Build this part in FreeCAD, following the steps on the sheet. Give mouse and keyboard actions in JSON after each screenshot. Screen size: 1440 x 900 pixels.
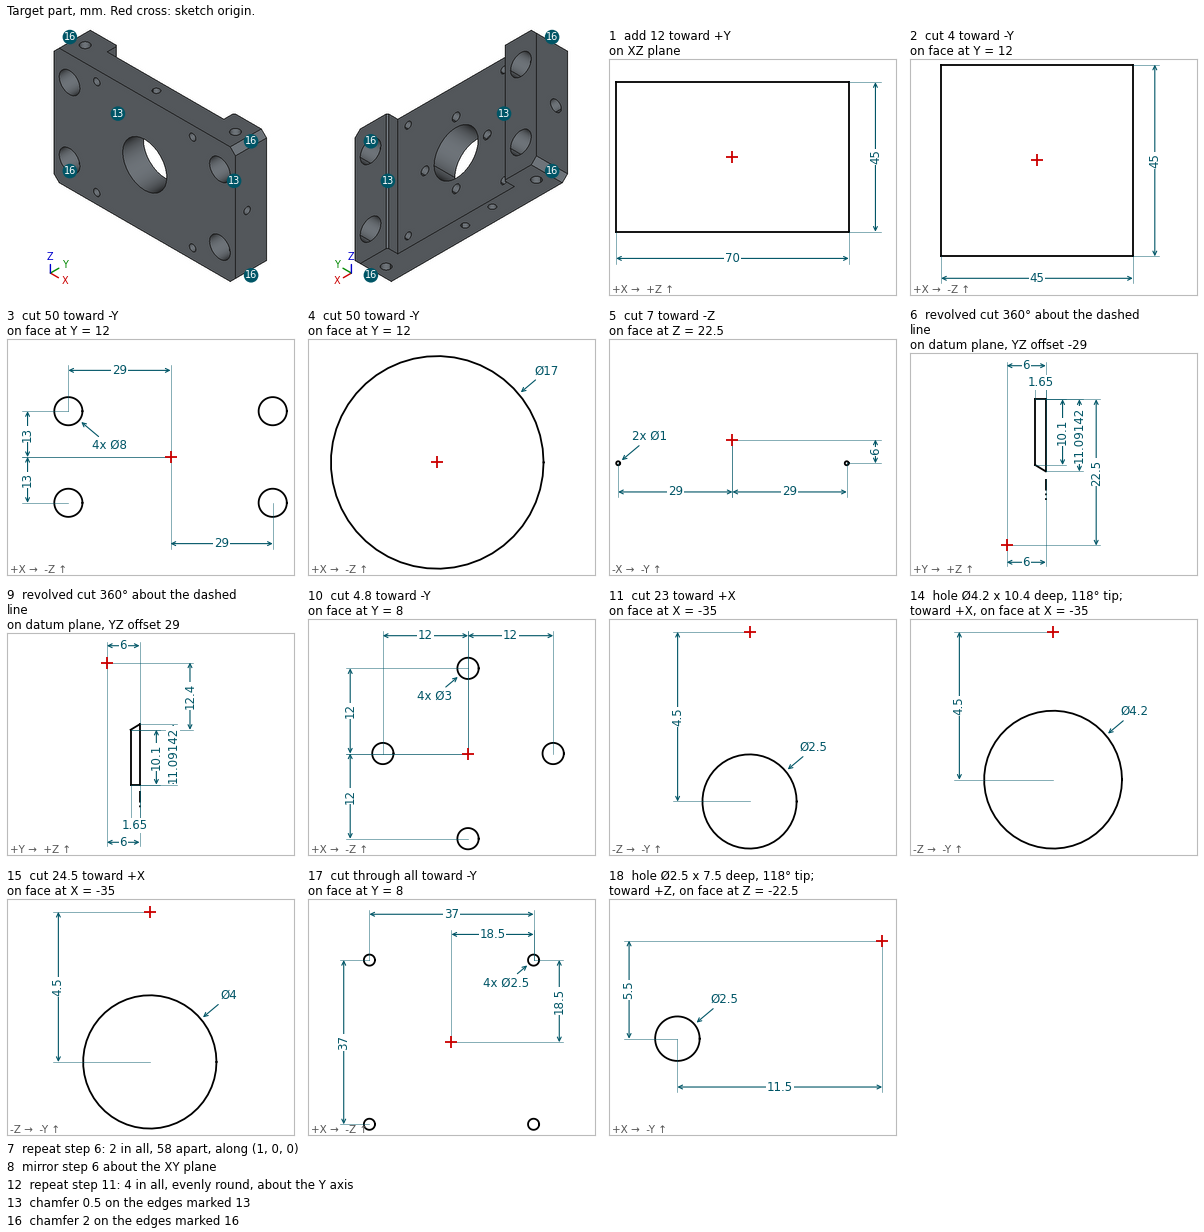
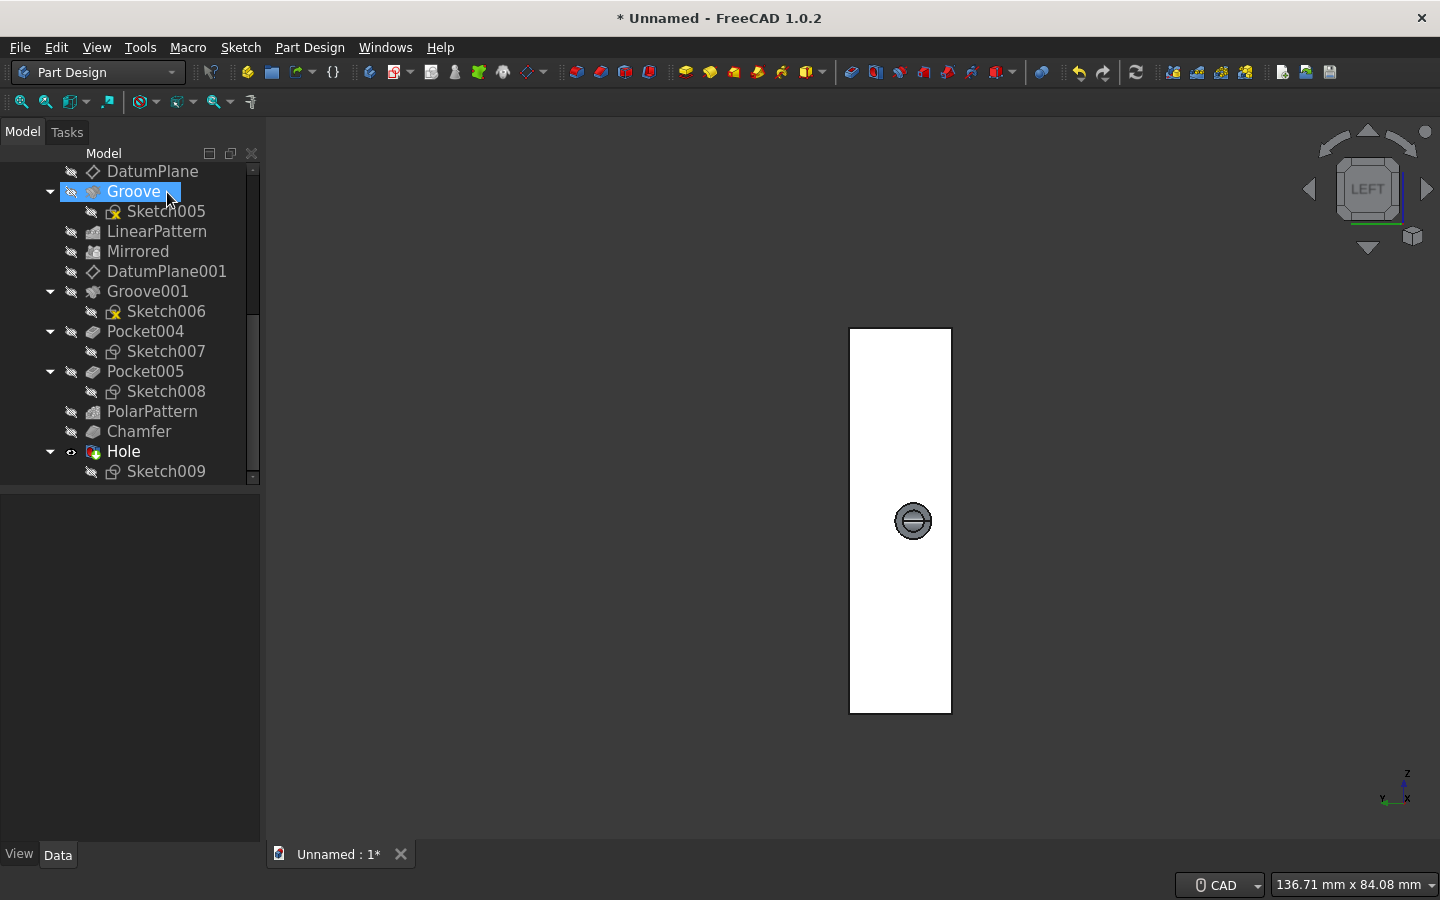
{"action": "left_click", "coordinate": [900, 410]}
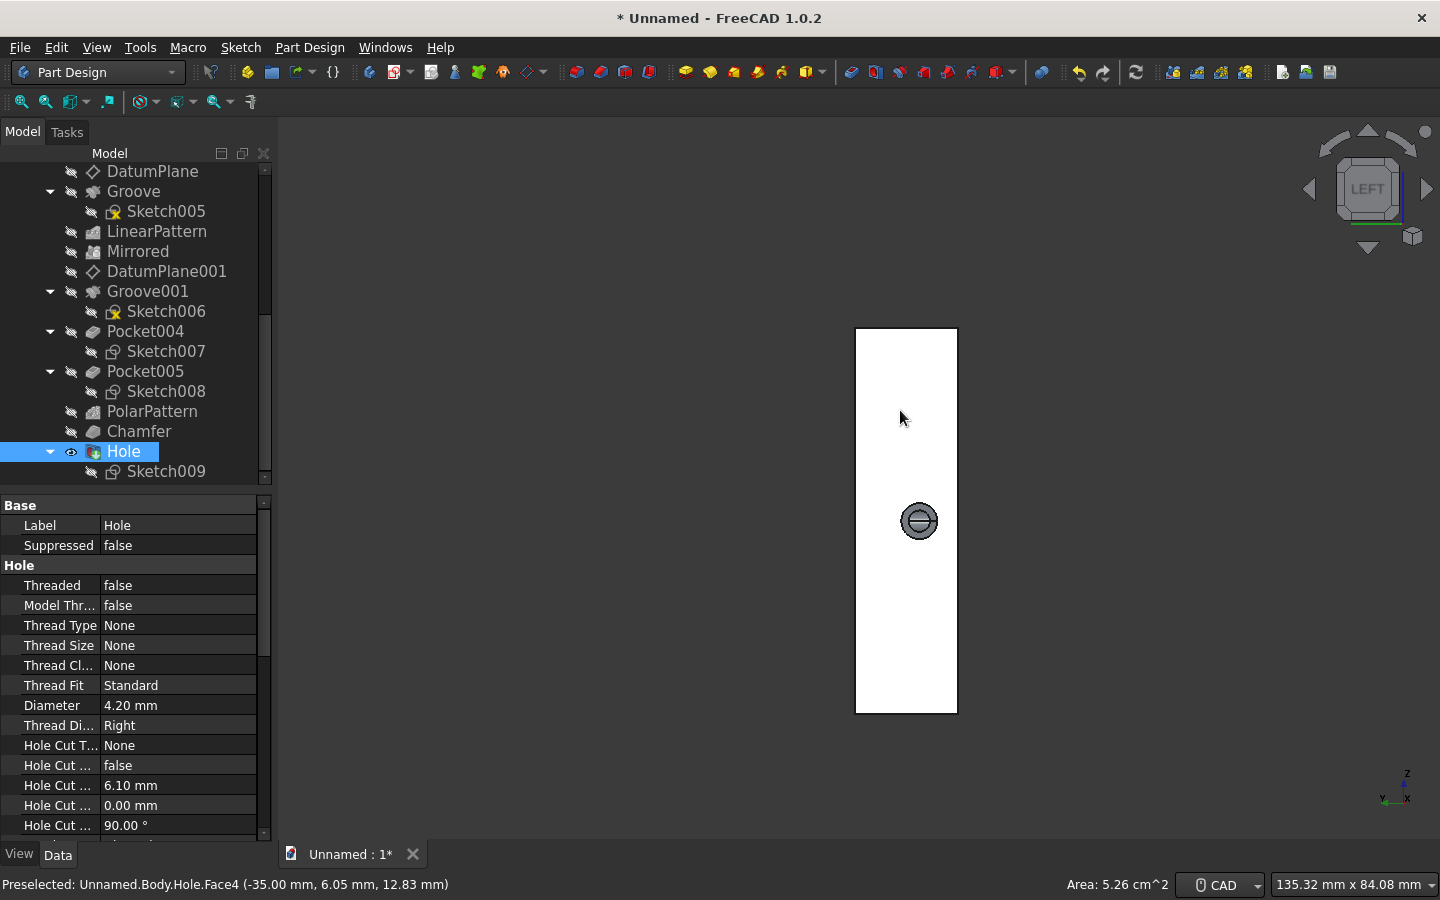
{"action": "left_click", "coordinate": [394, 72]}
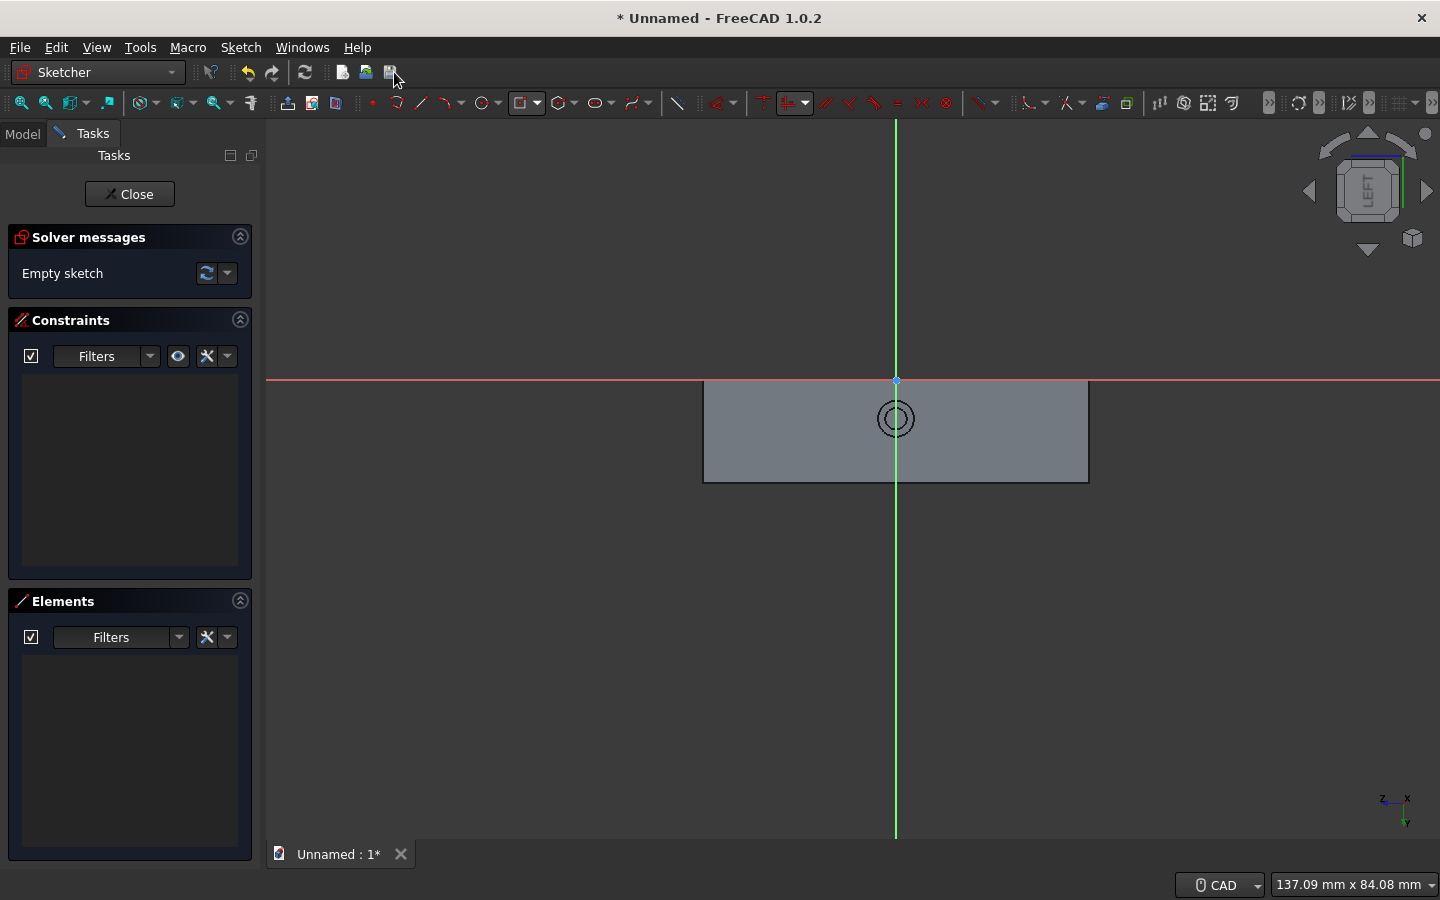
{"action": "scroll", "coordinate": [910, 399], "scroll_direction": "up", "scroll_amount": 11}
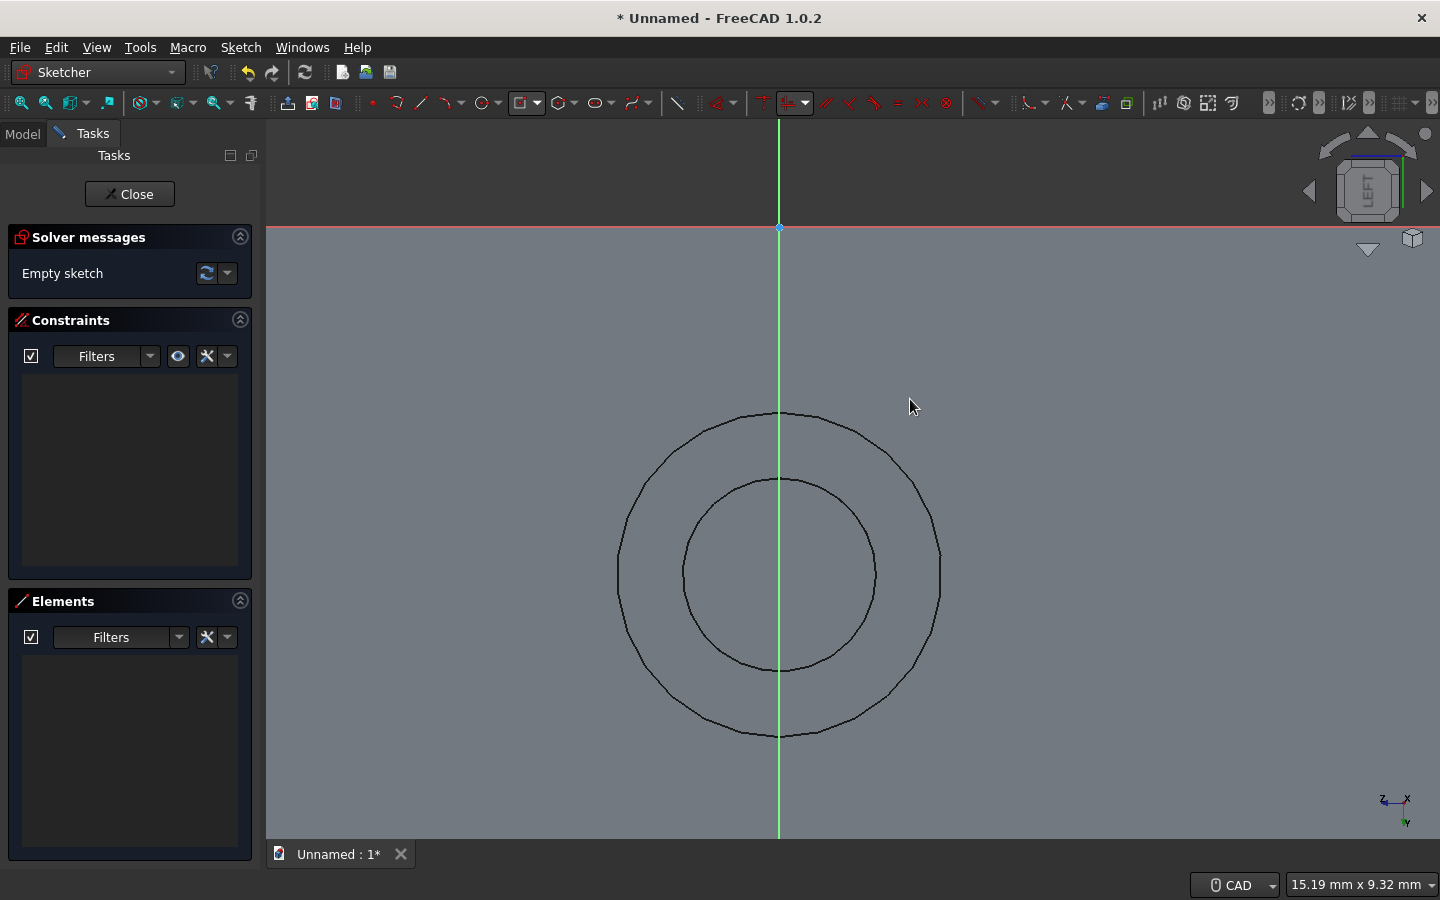
{"action": "left_click", "coordinate": [482, 104]}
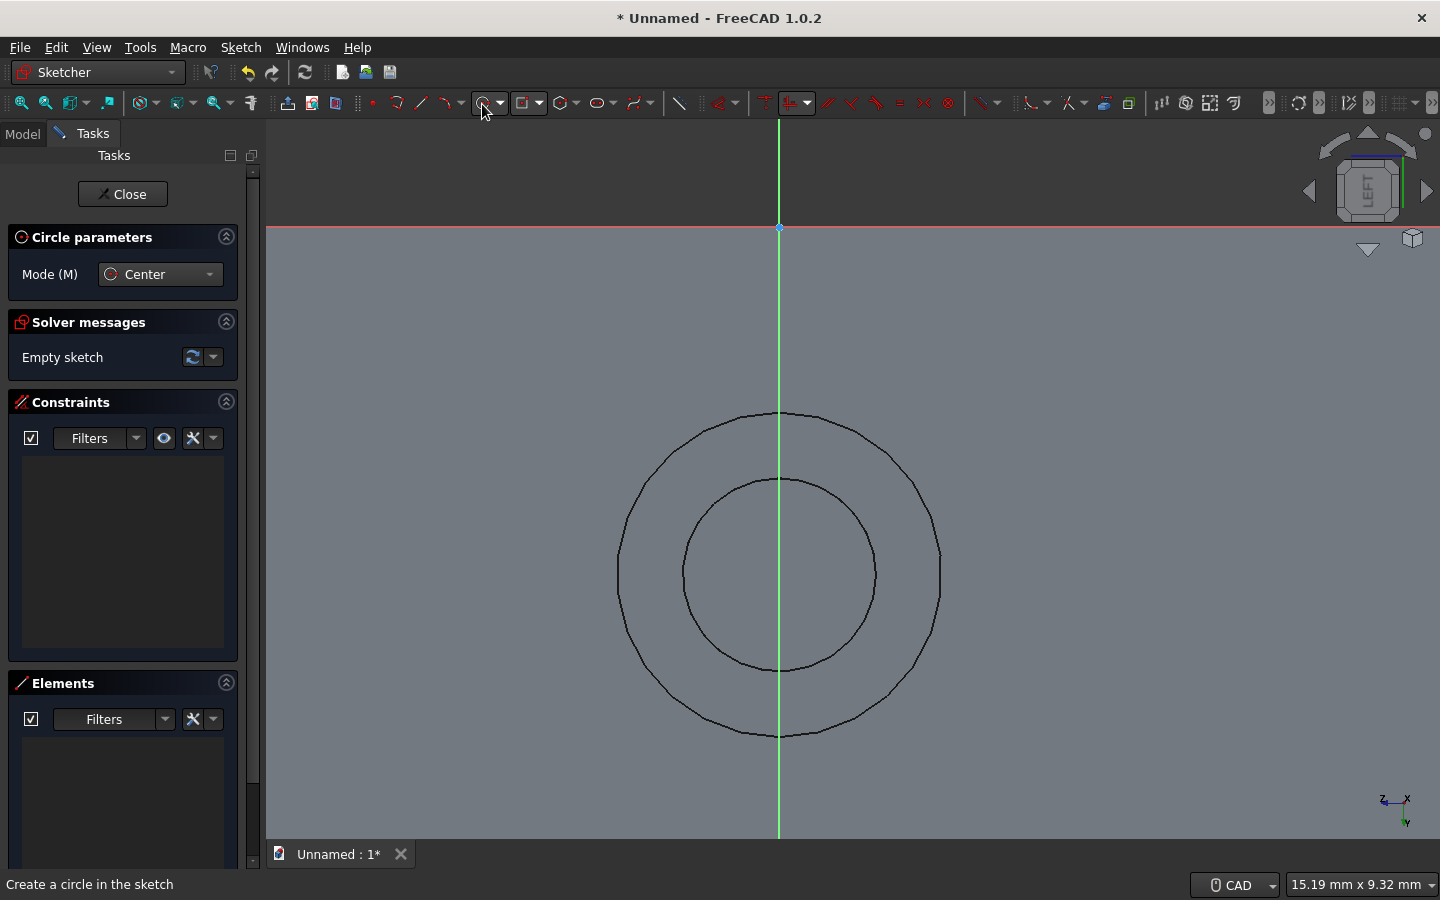
{"action": "left_click", "coordinate": [779, 575]}
{"action": "mouse_move", "coordinate": [889, 466]}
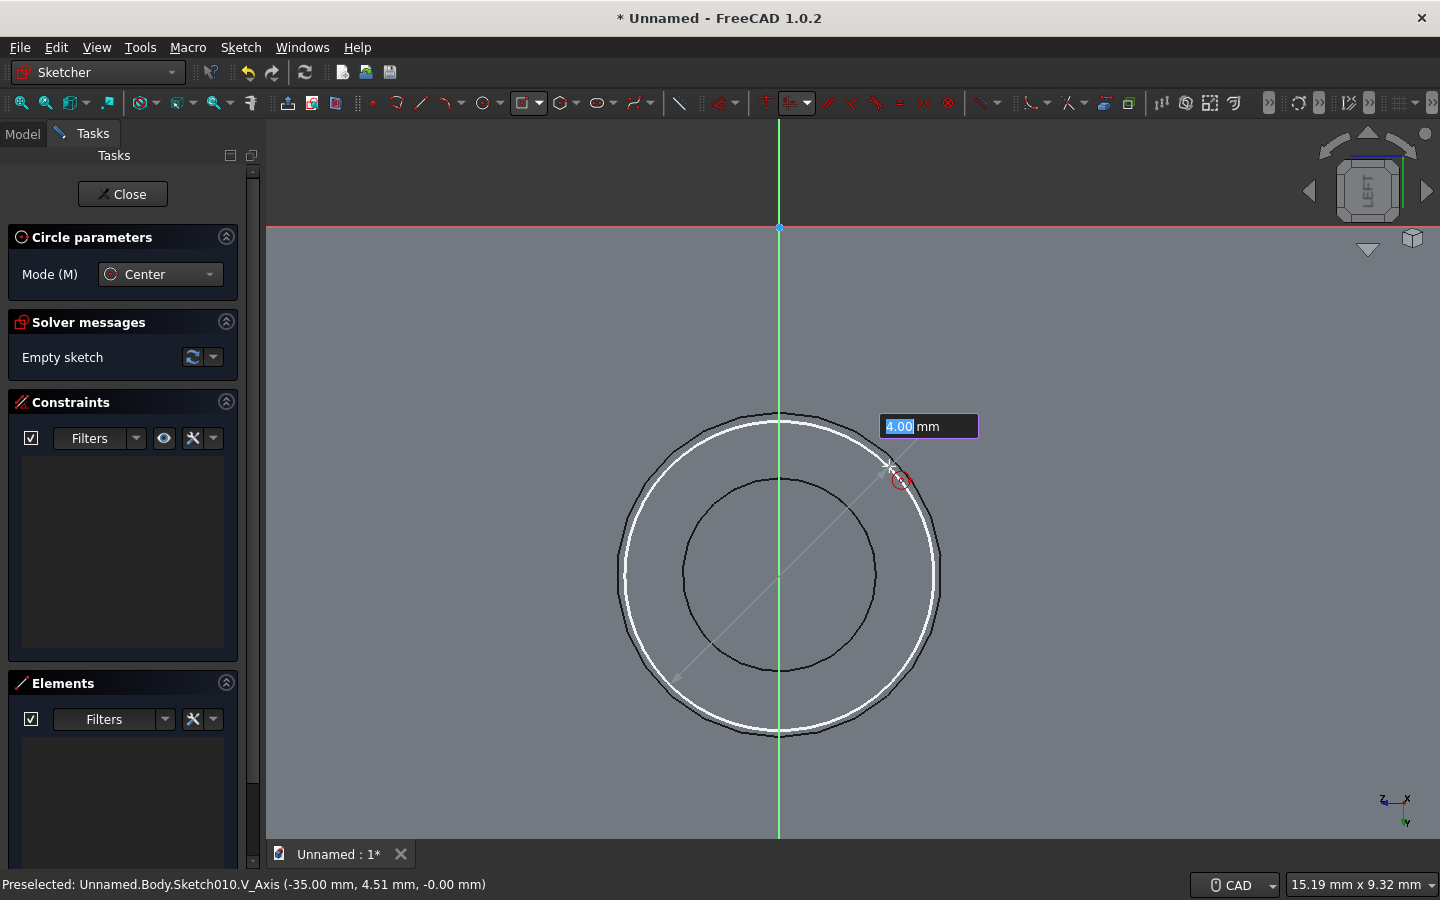
{"action": "type", "text": "4"}
{"action": "key", "text": "Return"}
{"action": "key", "text": "Escape"}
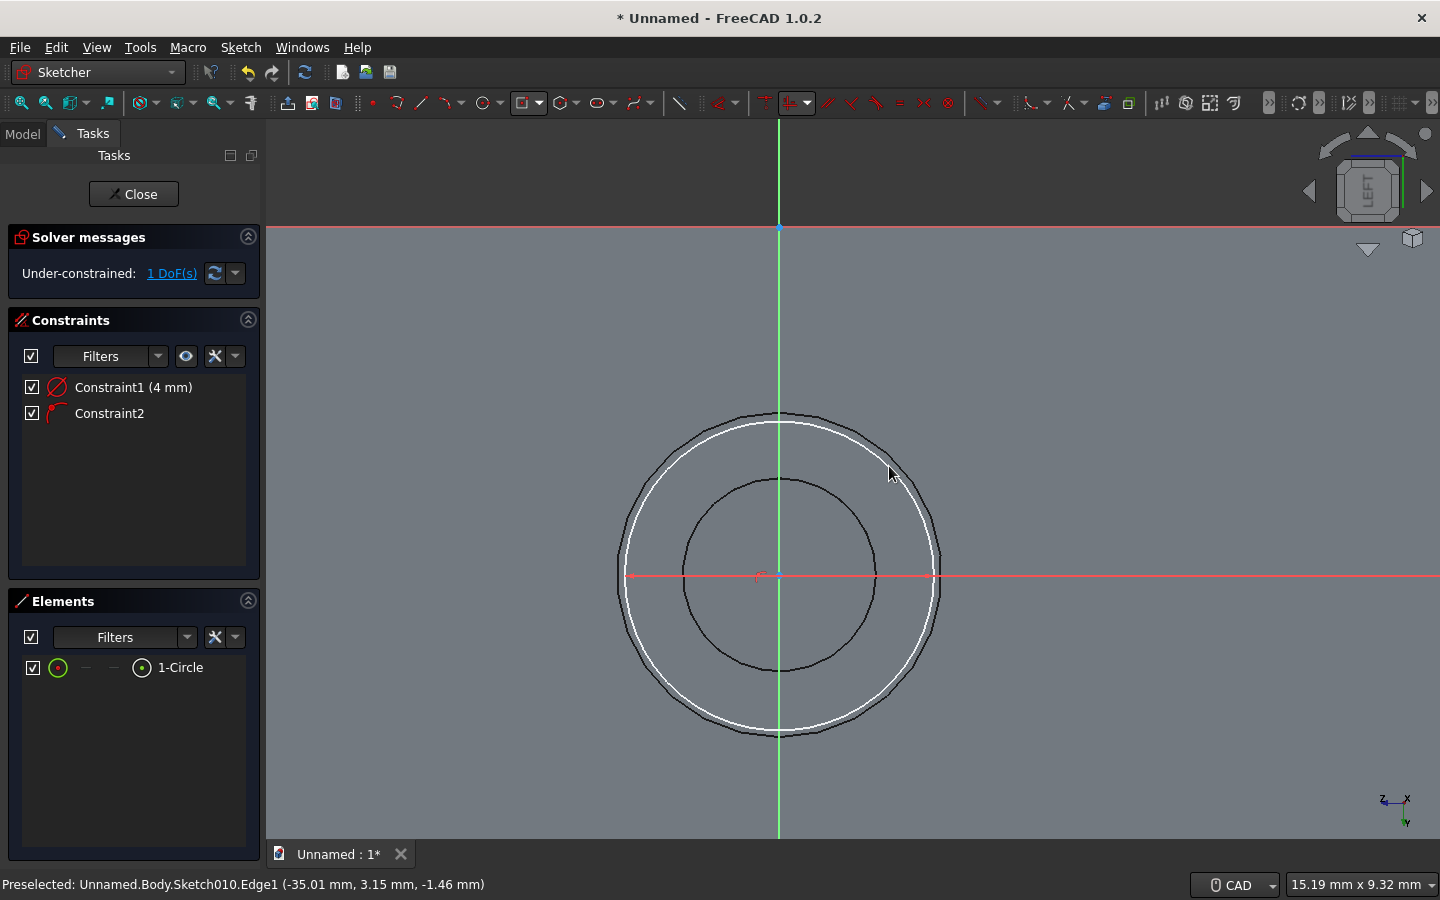
{"action": "left_click", "coordinate": [718, 104]}